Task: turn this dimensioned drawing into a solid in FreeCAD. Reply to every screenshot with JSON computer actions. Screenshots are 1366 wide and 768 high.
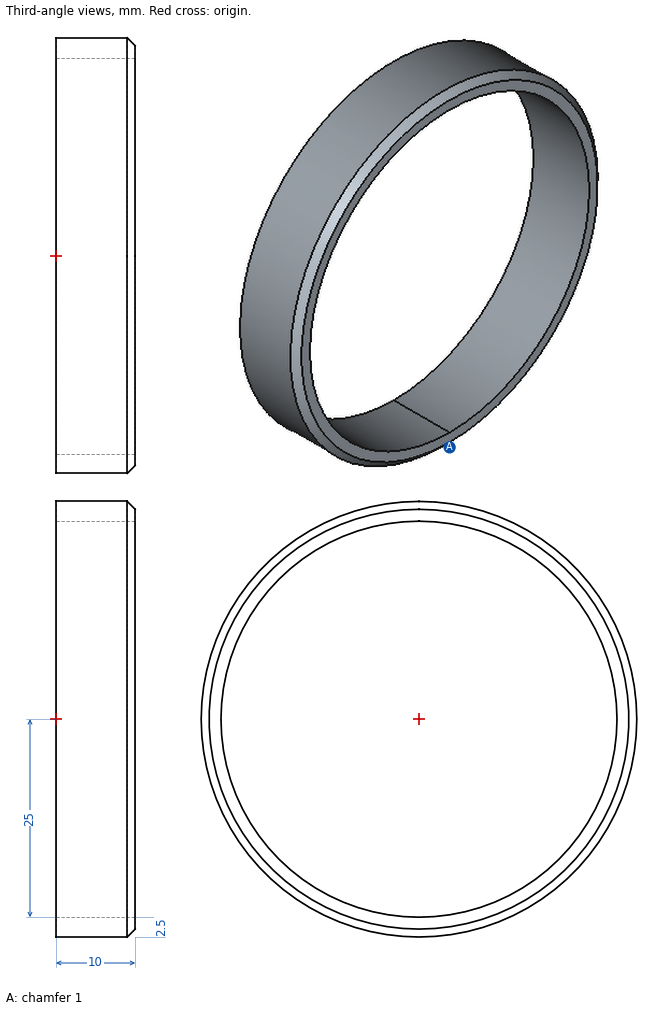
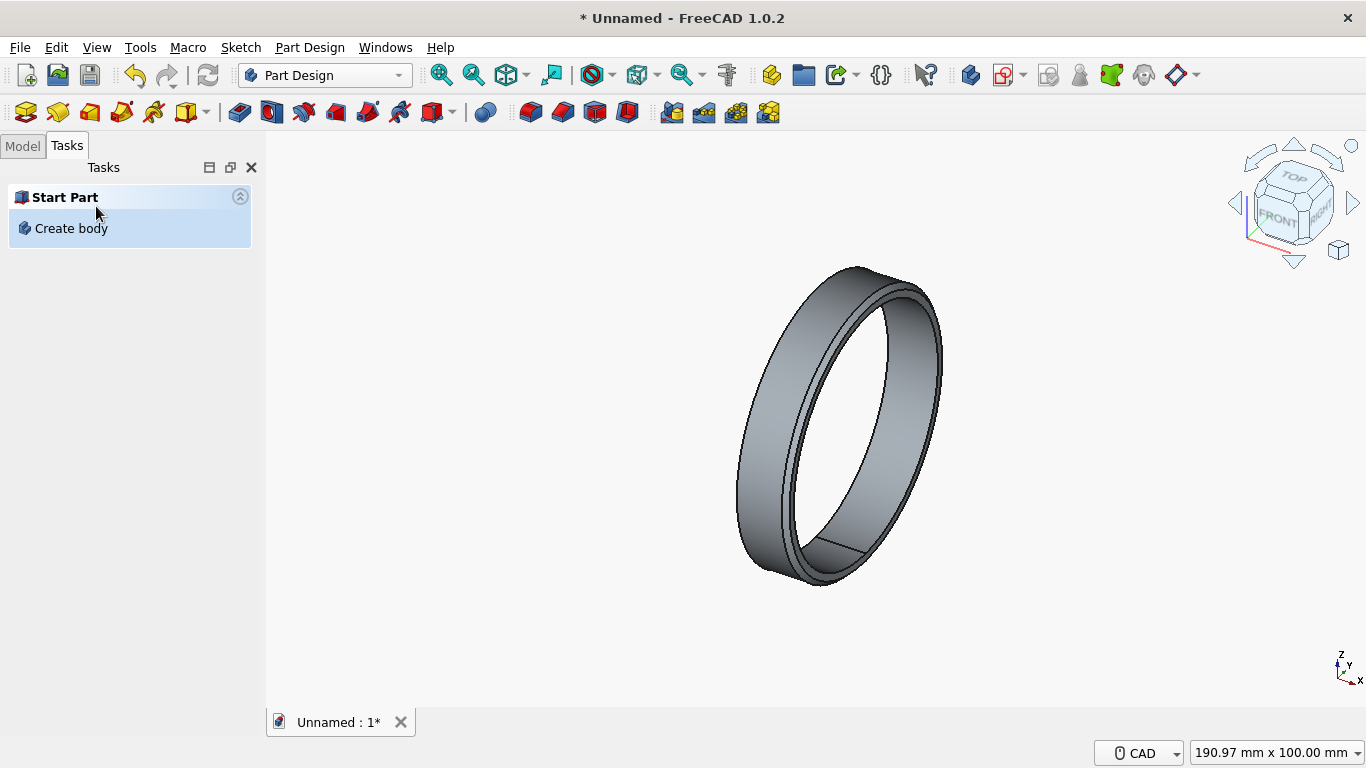
{"action": "key", "text": "0"}